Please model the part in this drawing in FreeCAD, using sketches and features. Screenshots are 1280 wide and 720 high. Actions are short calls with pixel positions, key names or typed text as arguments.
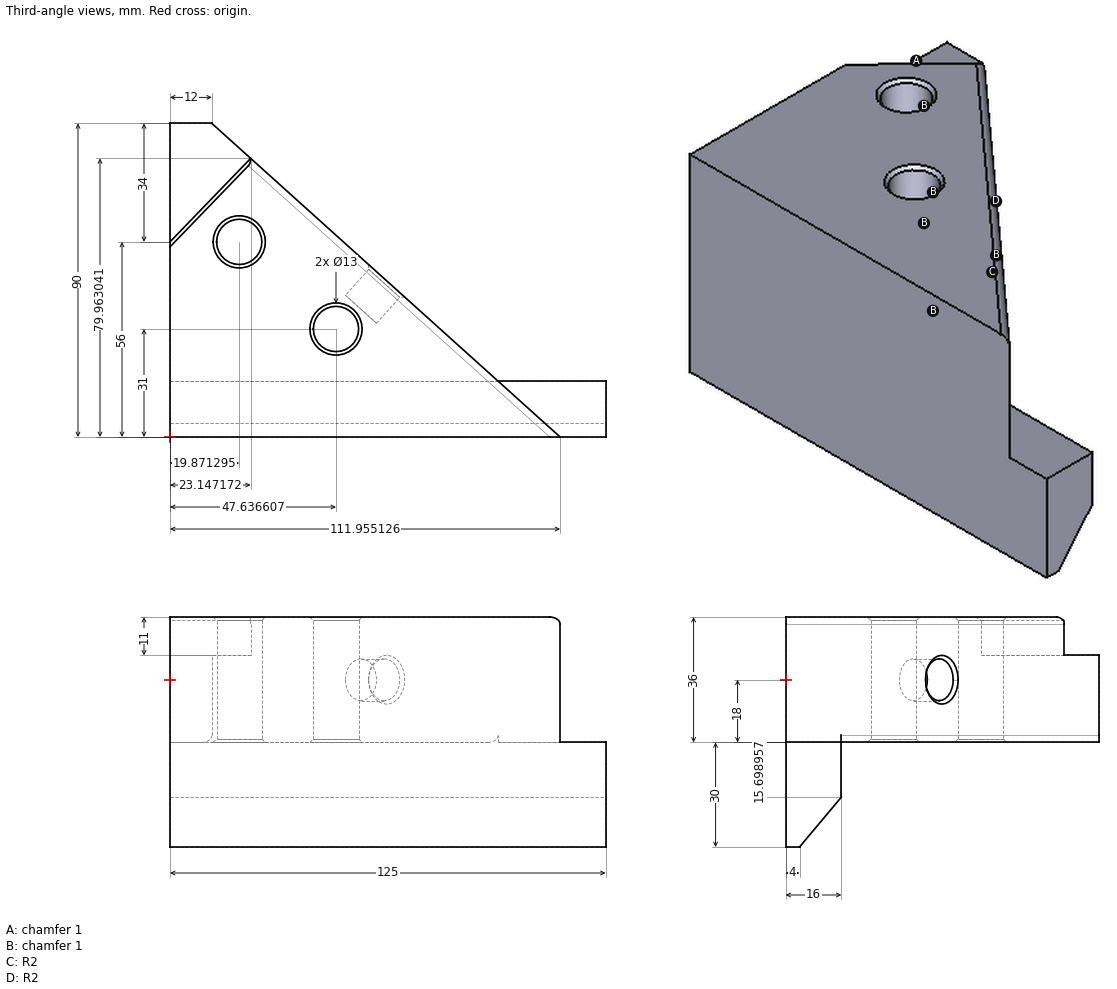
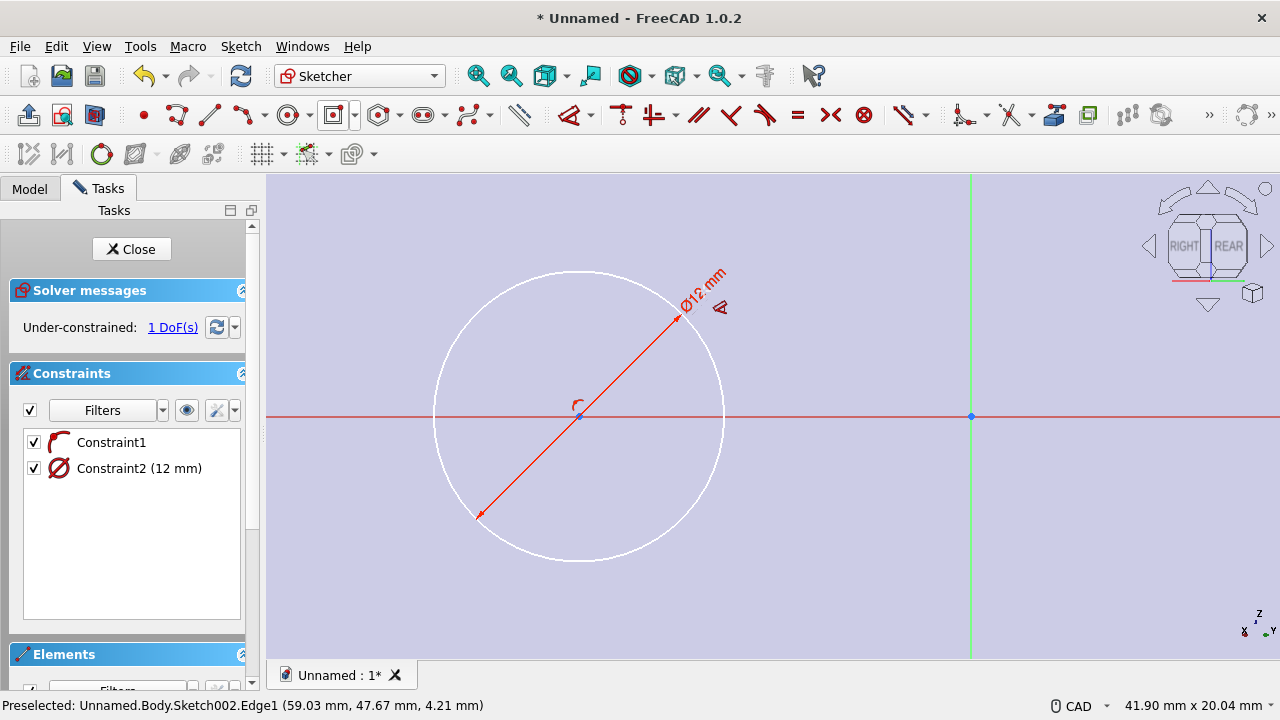
click(579, 416)
click(775, 450)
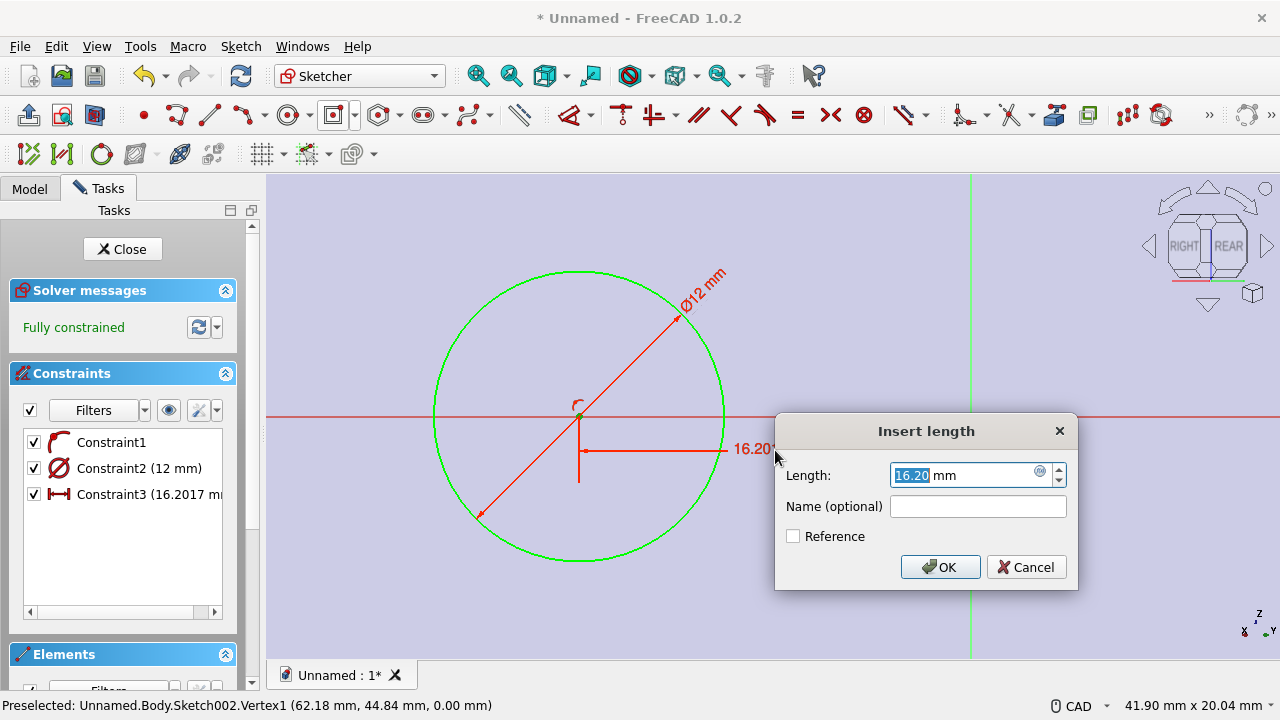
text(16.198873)
key(Return)
key(Escape)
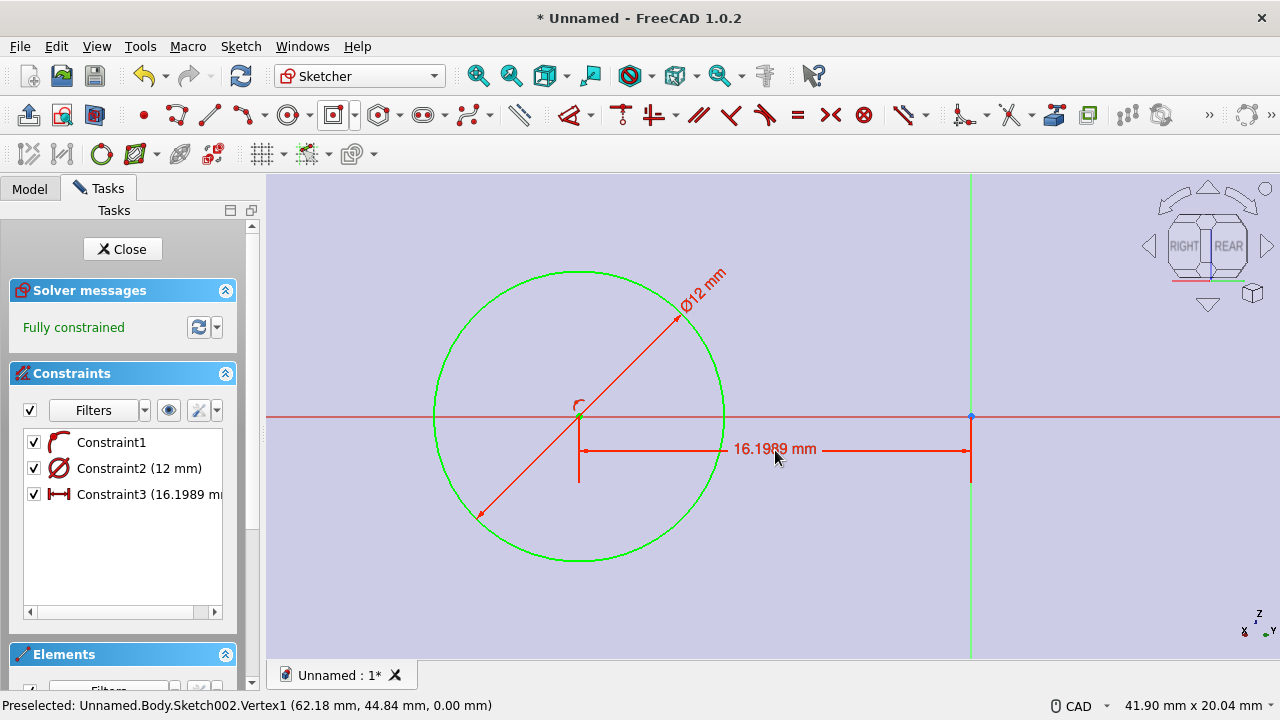
click(123, 249)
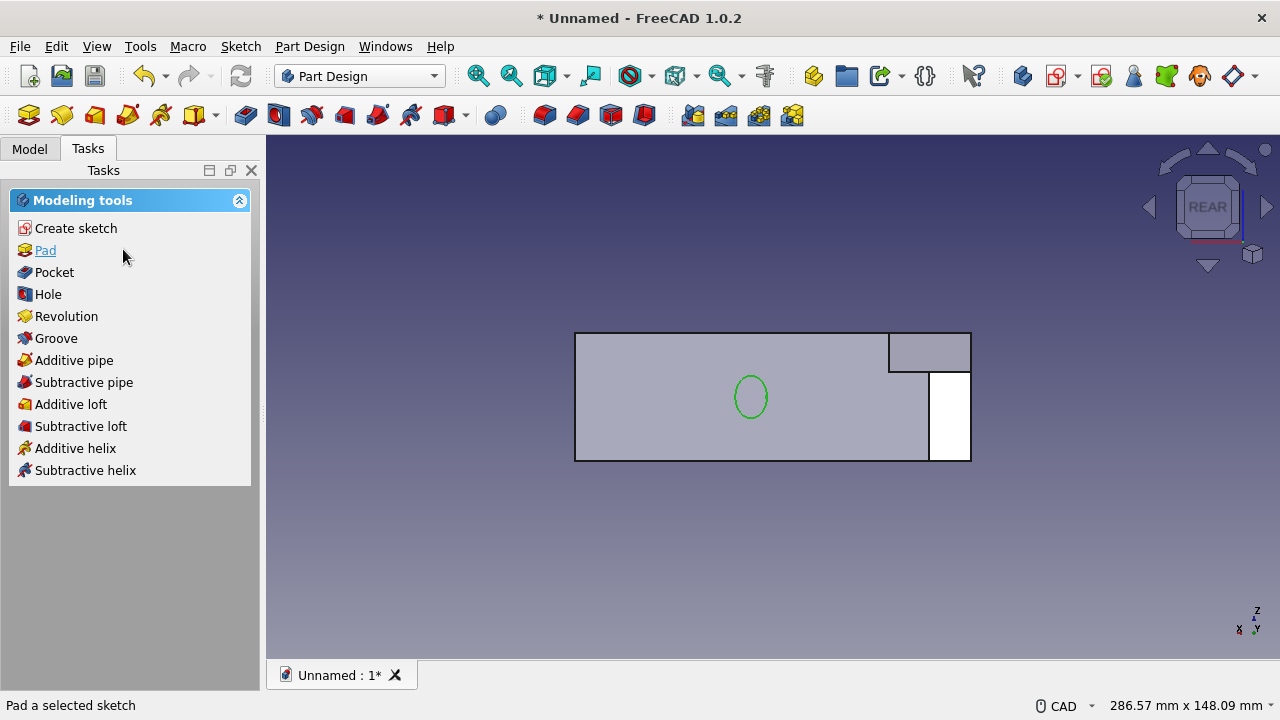
click(246, 116)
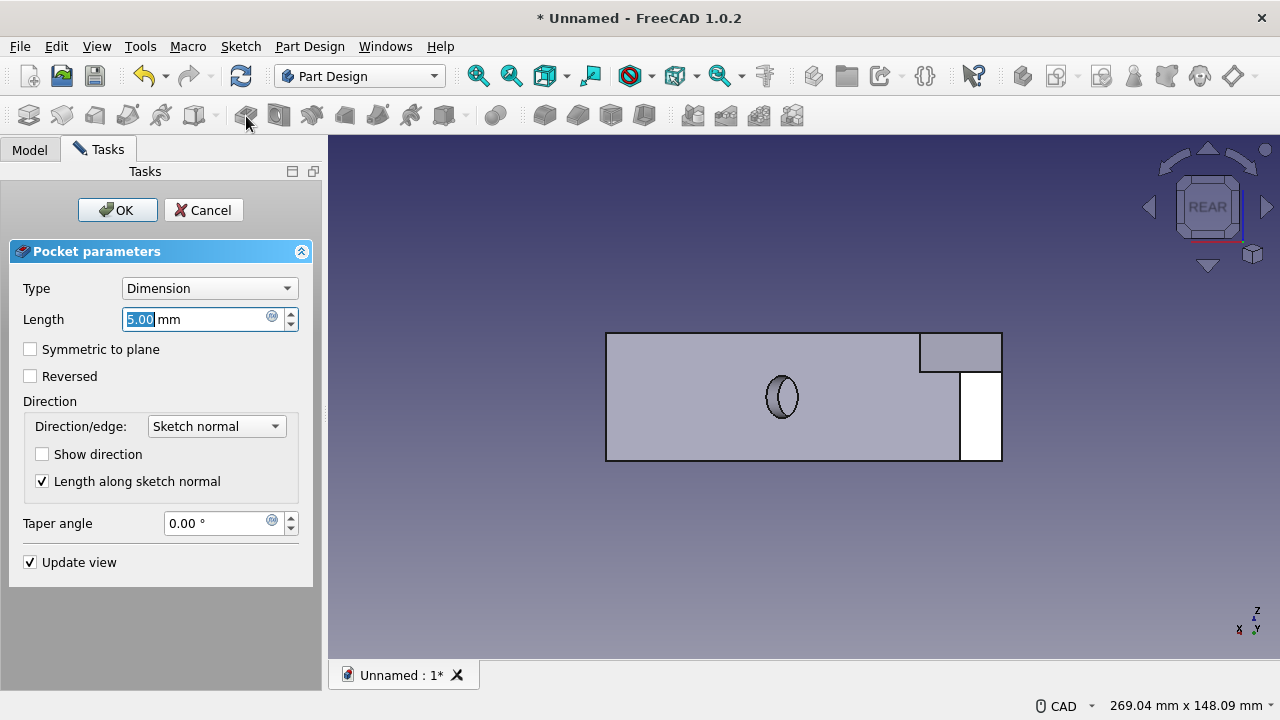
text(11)
key(Tab)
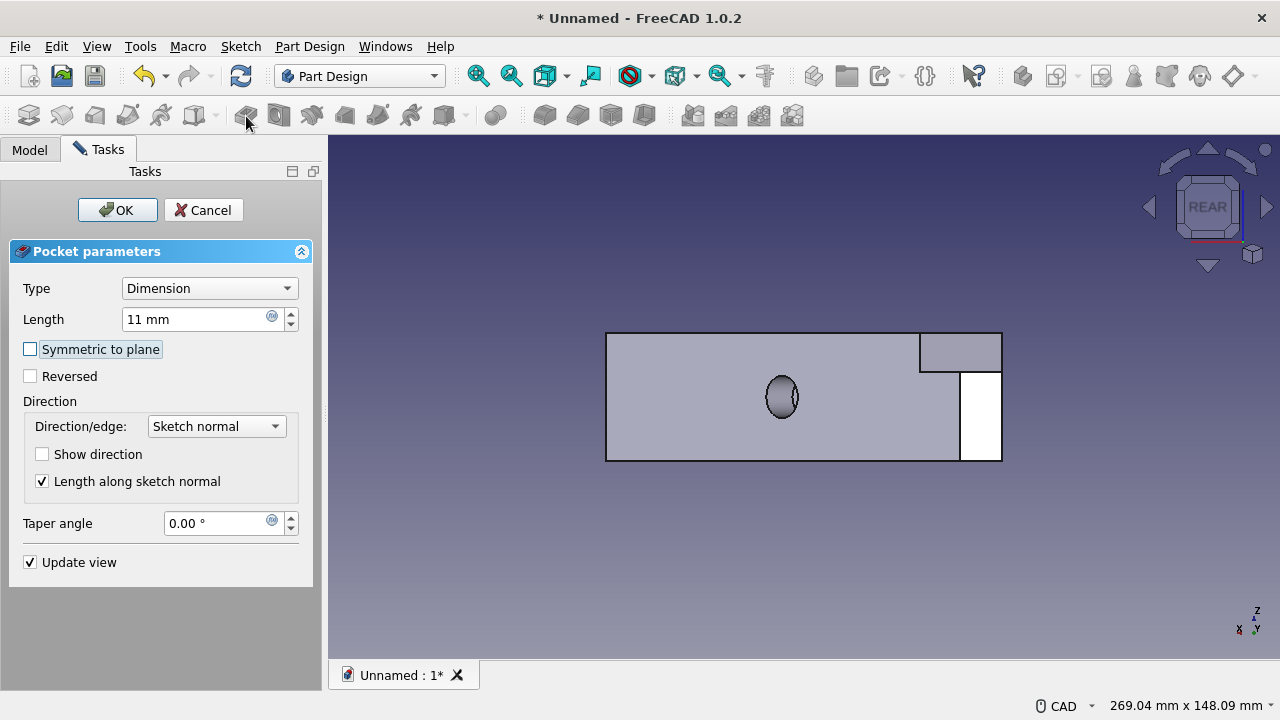
click(118, 210)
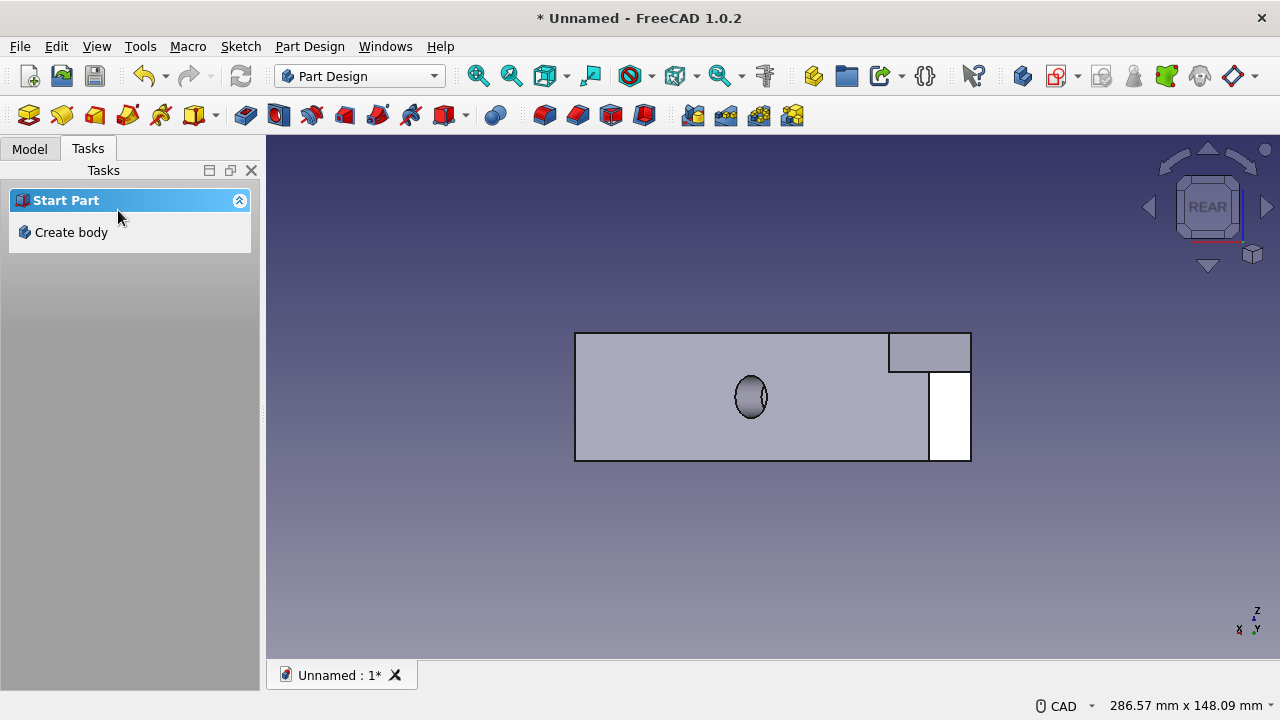
click(479, 76)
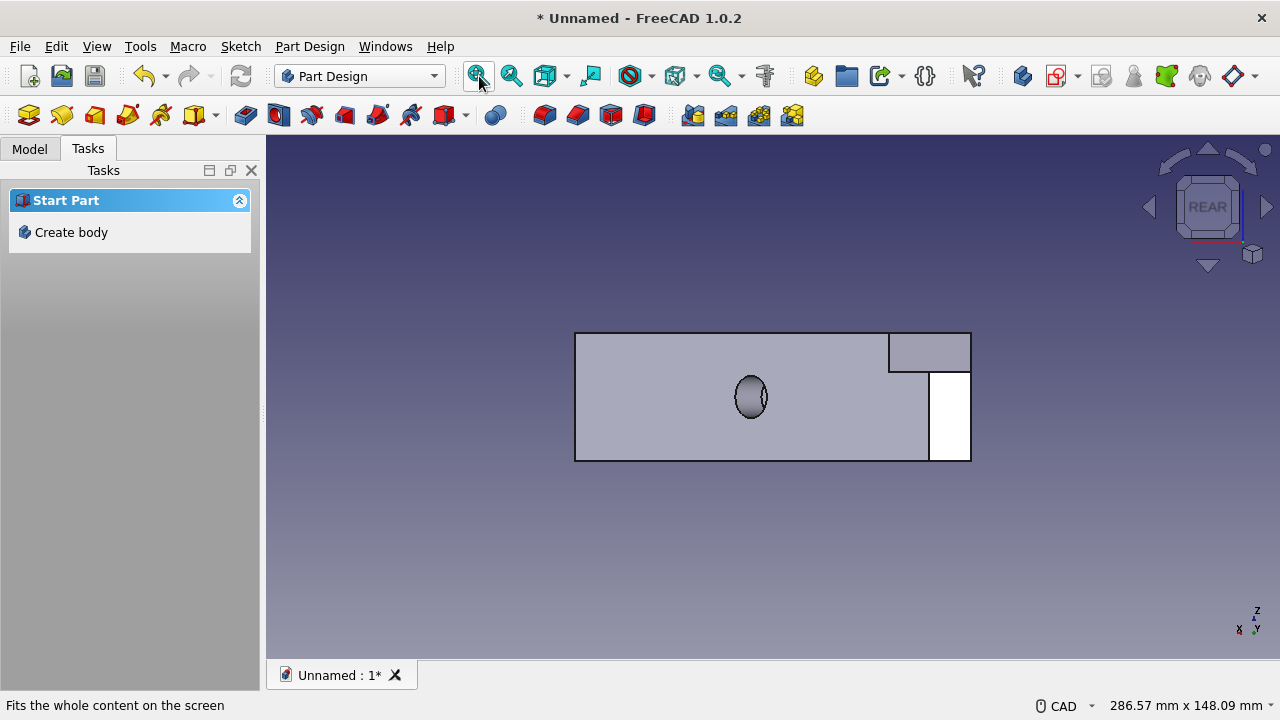
click(1056, 76)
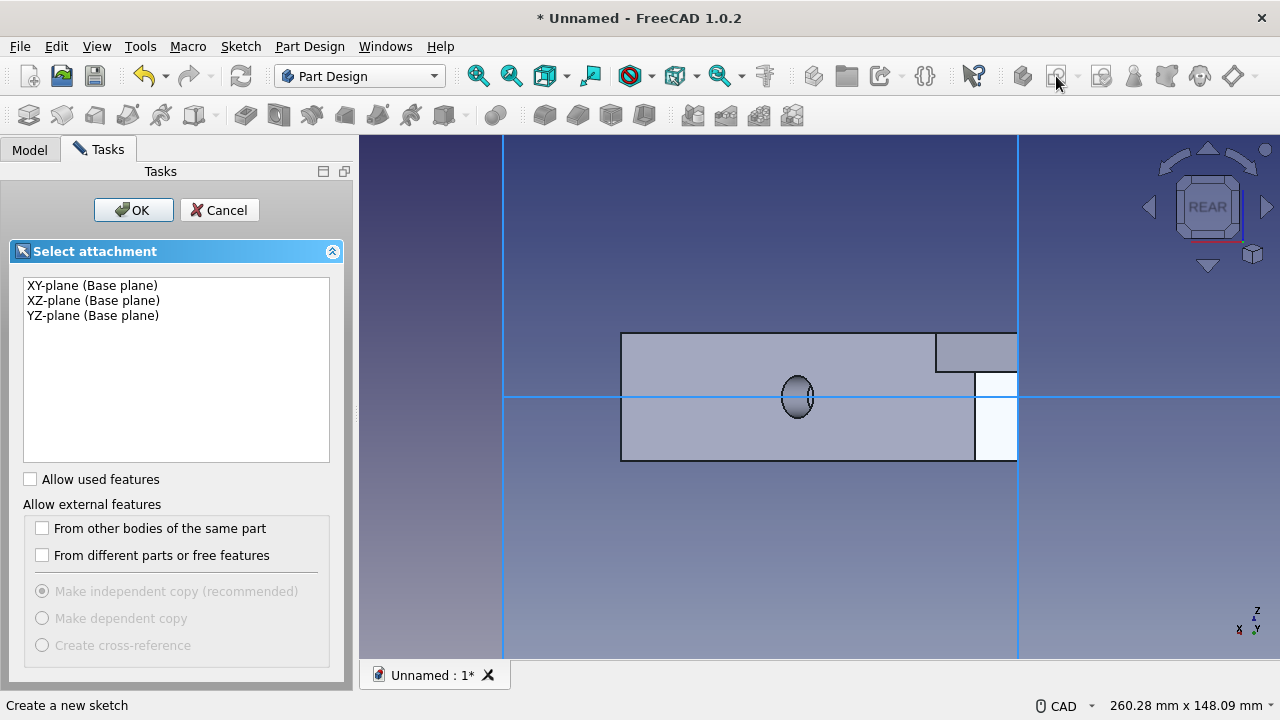
click(84, 316)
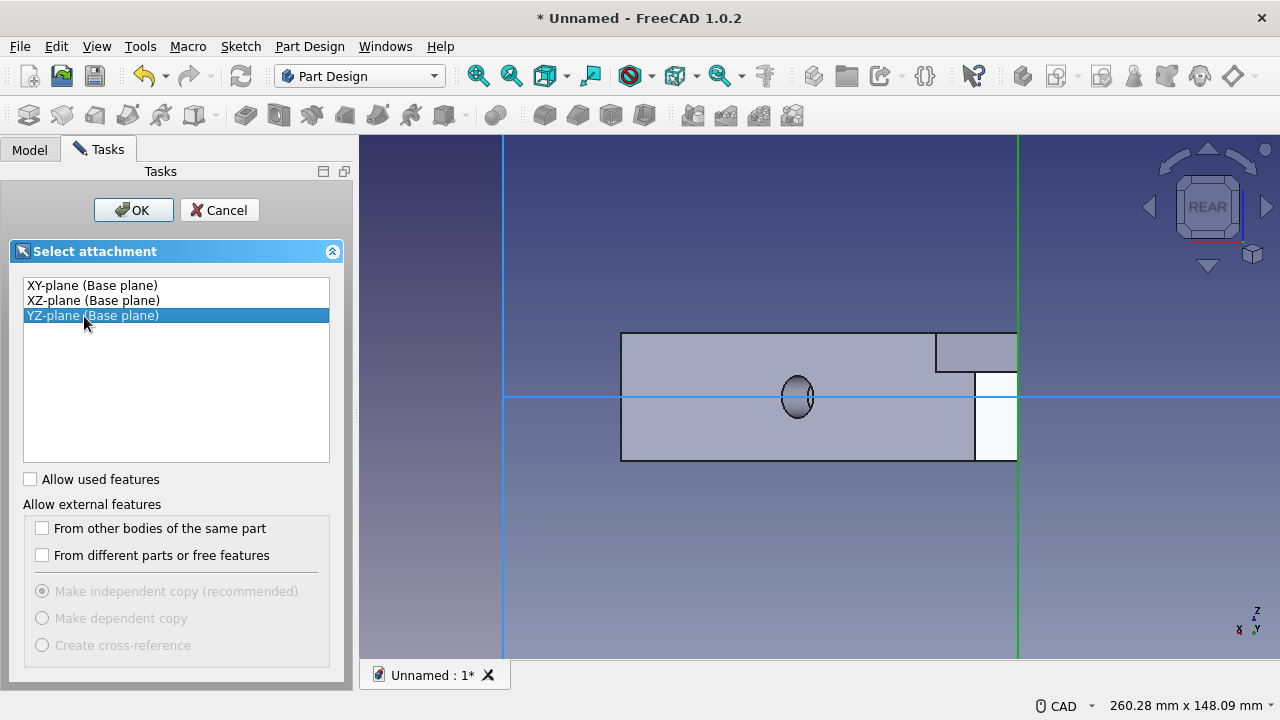
click(134, 210)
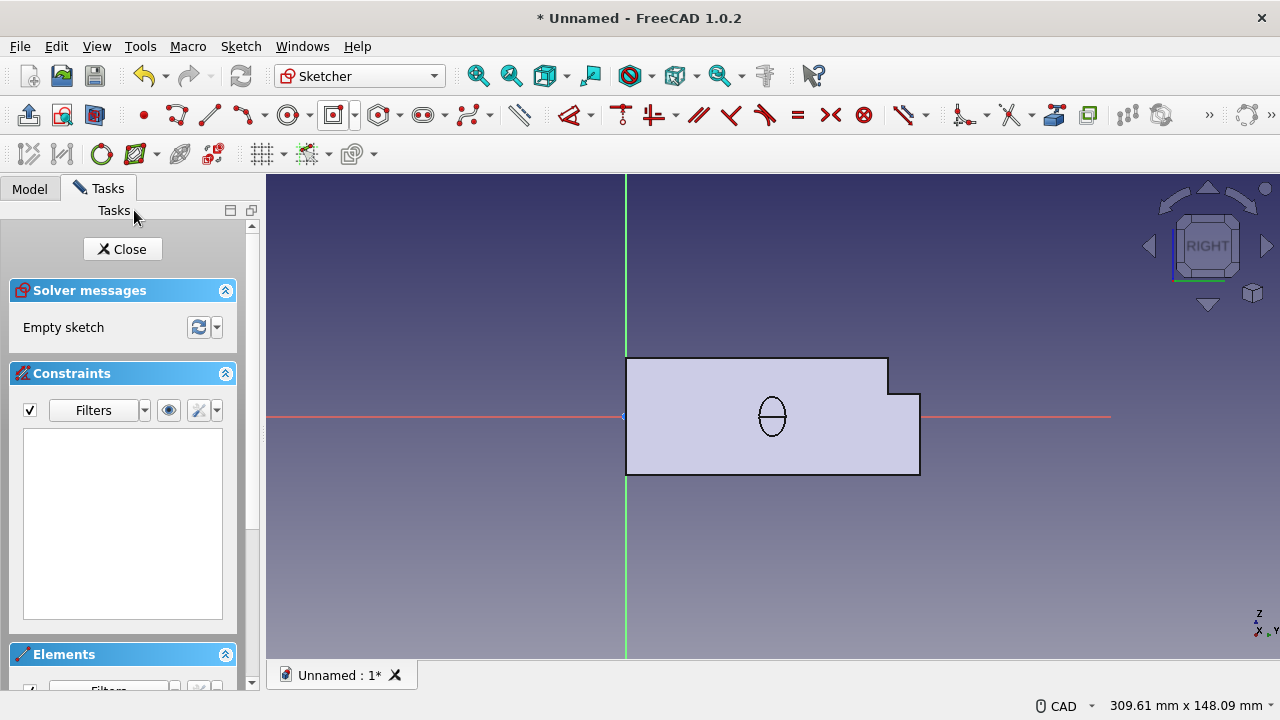
click(95, 116)